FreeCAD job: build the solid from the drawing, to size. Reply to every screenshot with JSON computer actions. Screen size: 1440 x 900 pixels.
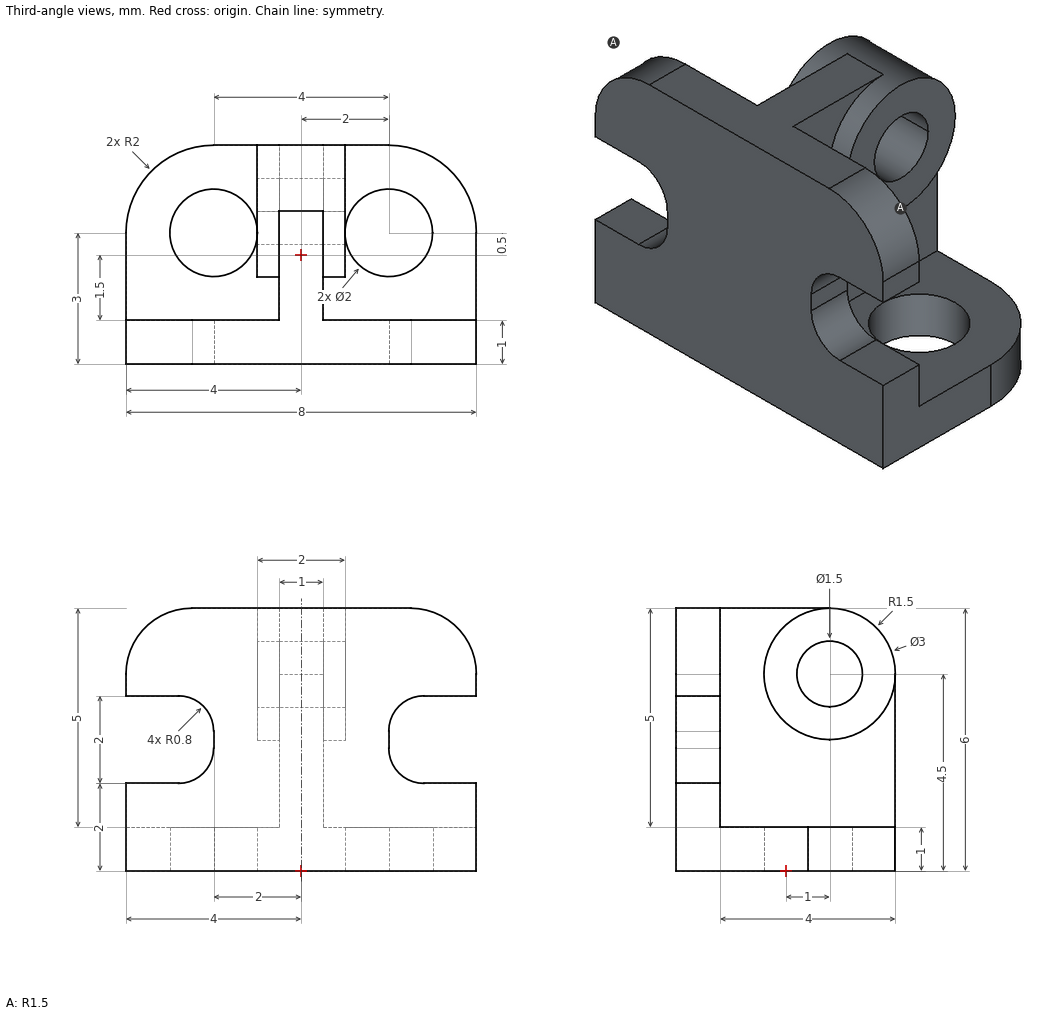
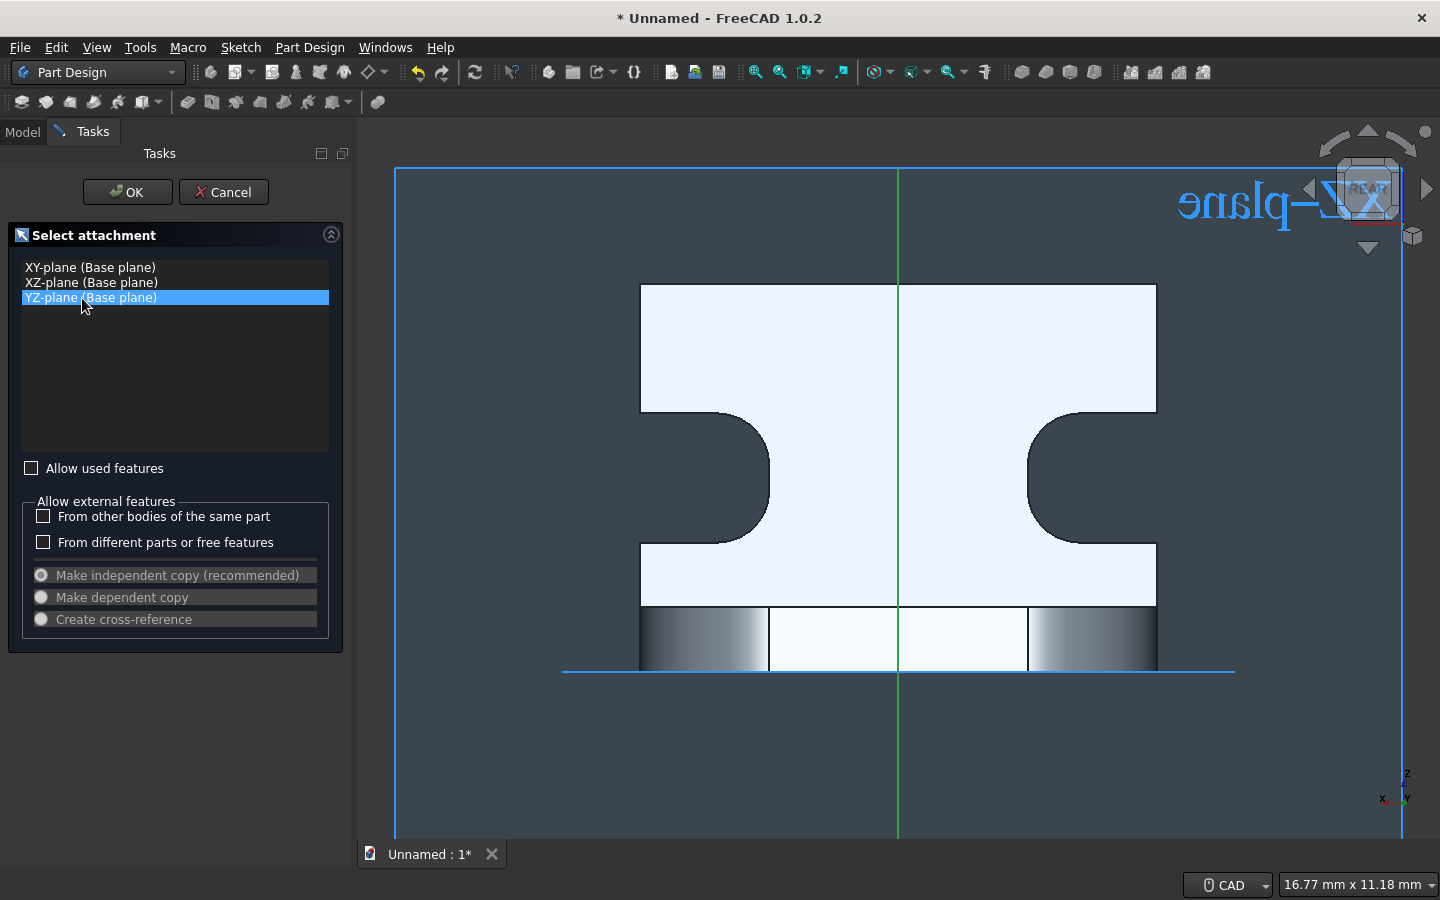
{"action": "left_click", "coordinate": [128, 192]}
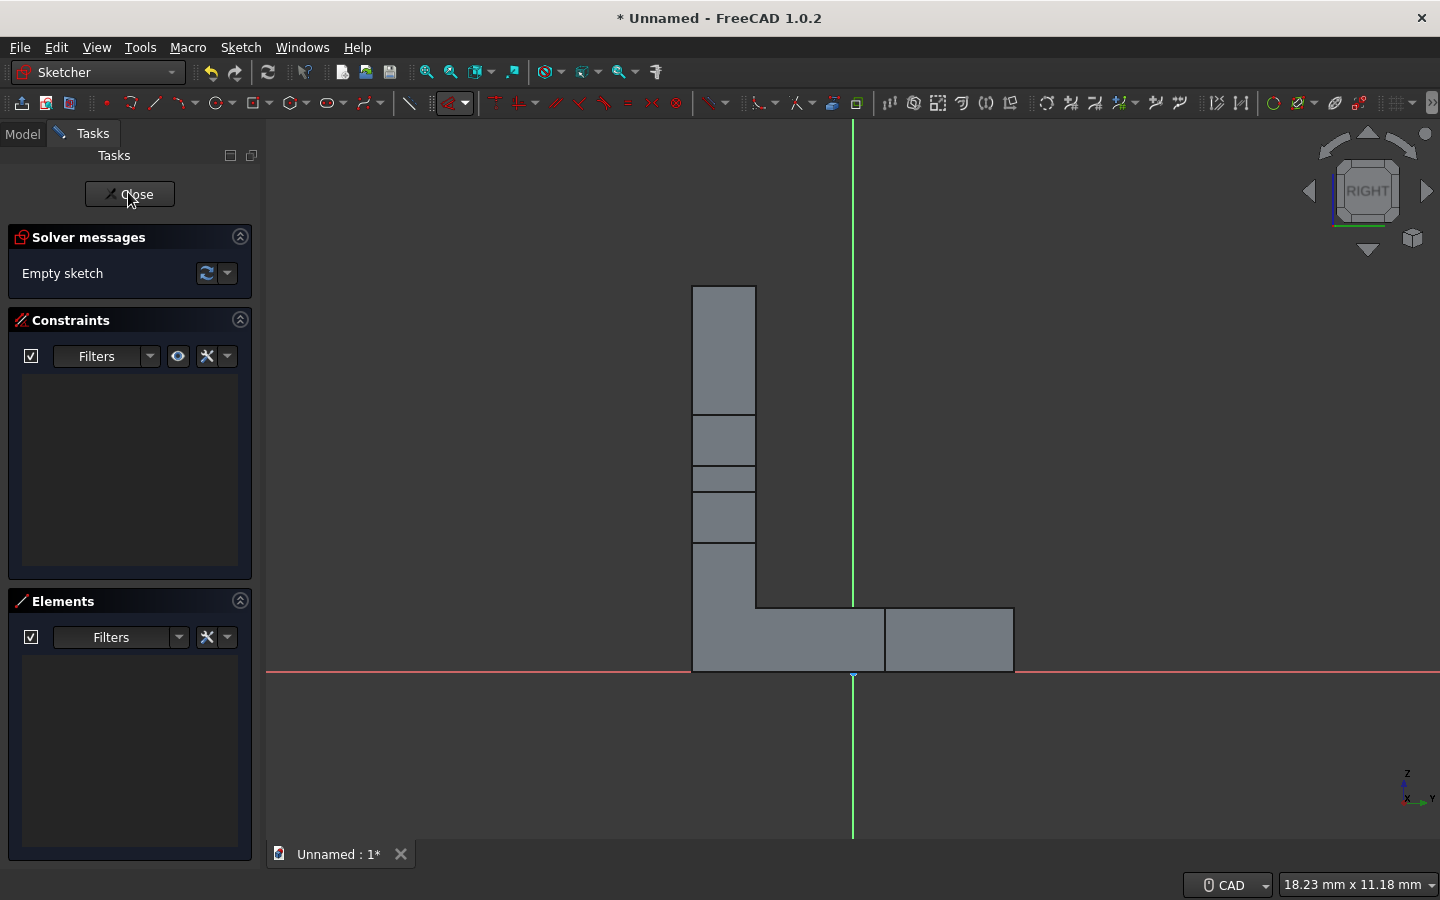
{"action": "left_click", "coordinate": [70, 104]}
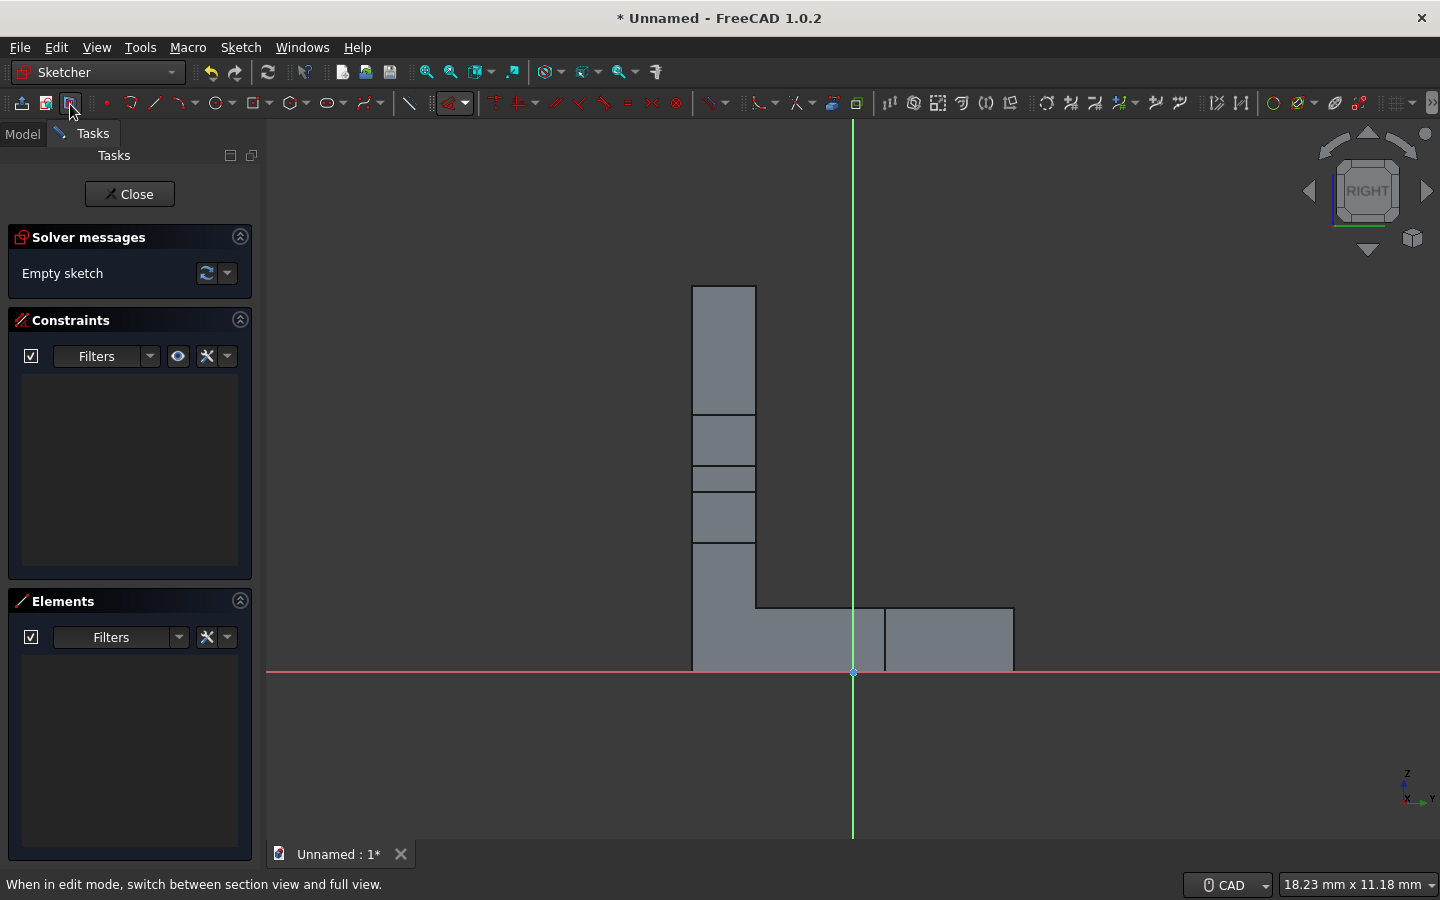
{"action": "left_click", "coordinate": [132, 104]}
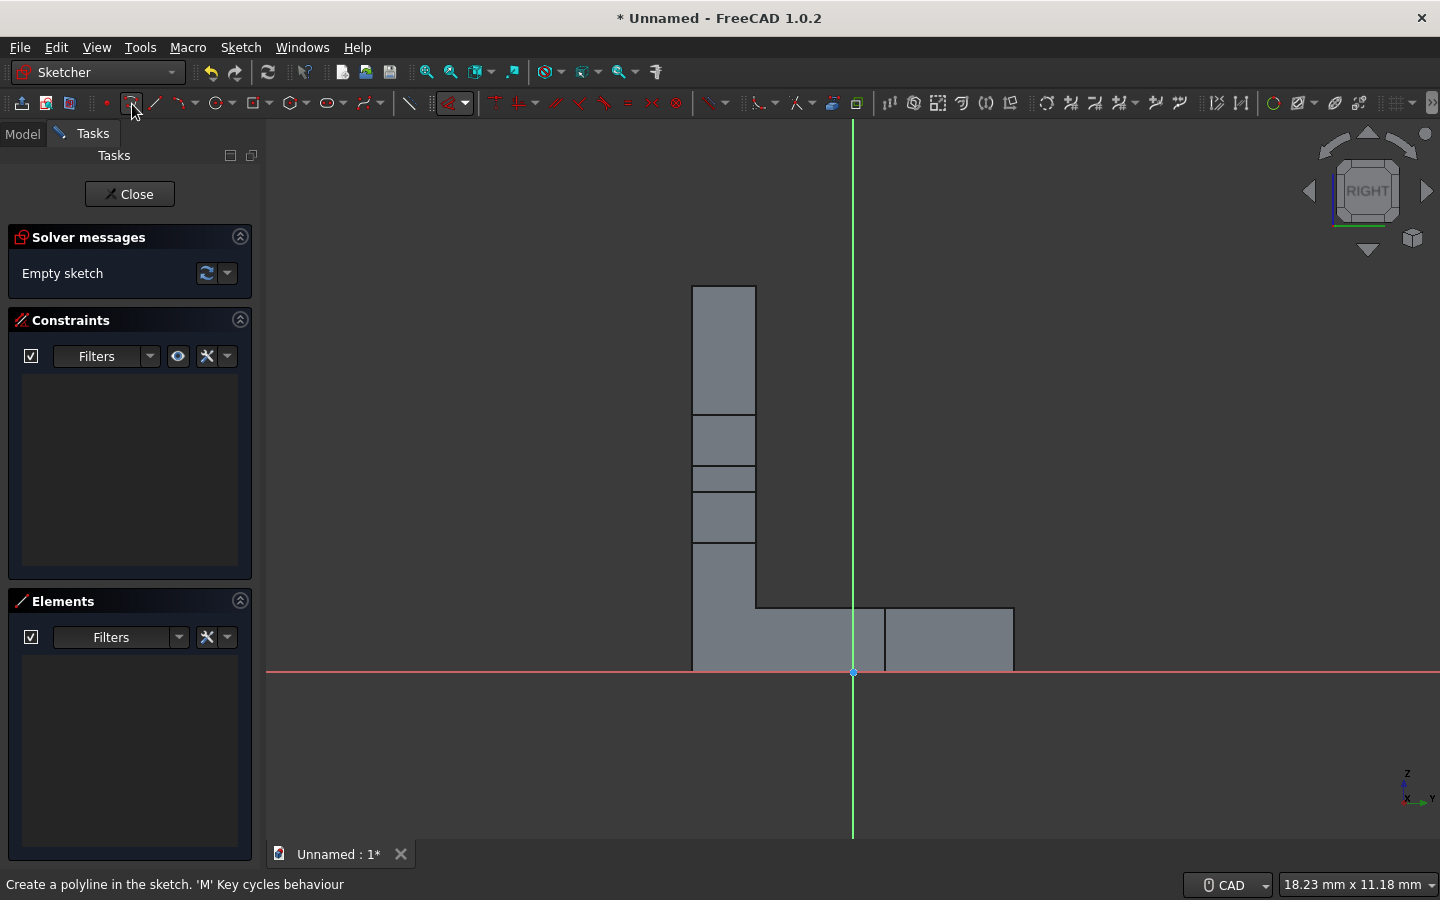
{"action": "left_click", "coordinate": [917, 286]}
{"action": "left_click", "coordinate": [756, 286]}
{"action": "left_click", "coordinate": [756, 608]}
{"action": "left_click", "coordinate": [1014, 608]}
{"action": "left_click", "coordinate": [1014, 382]}
{"action": "right_click", "coordinate": [1014, 382]}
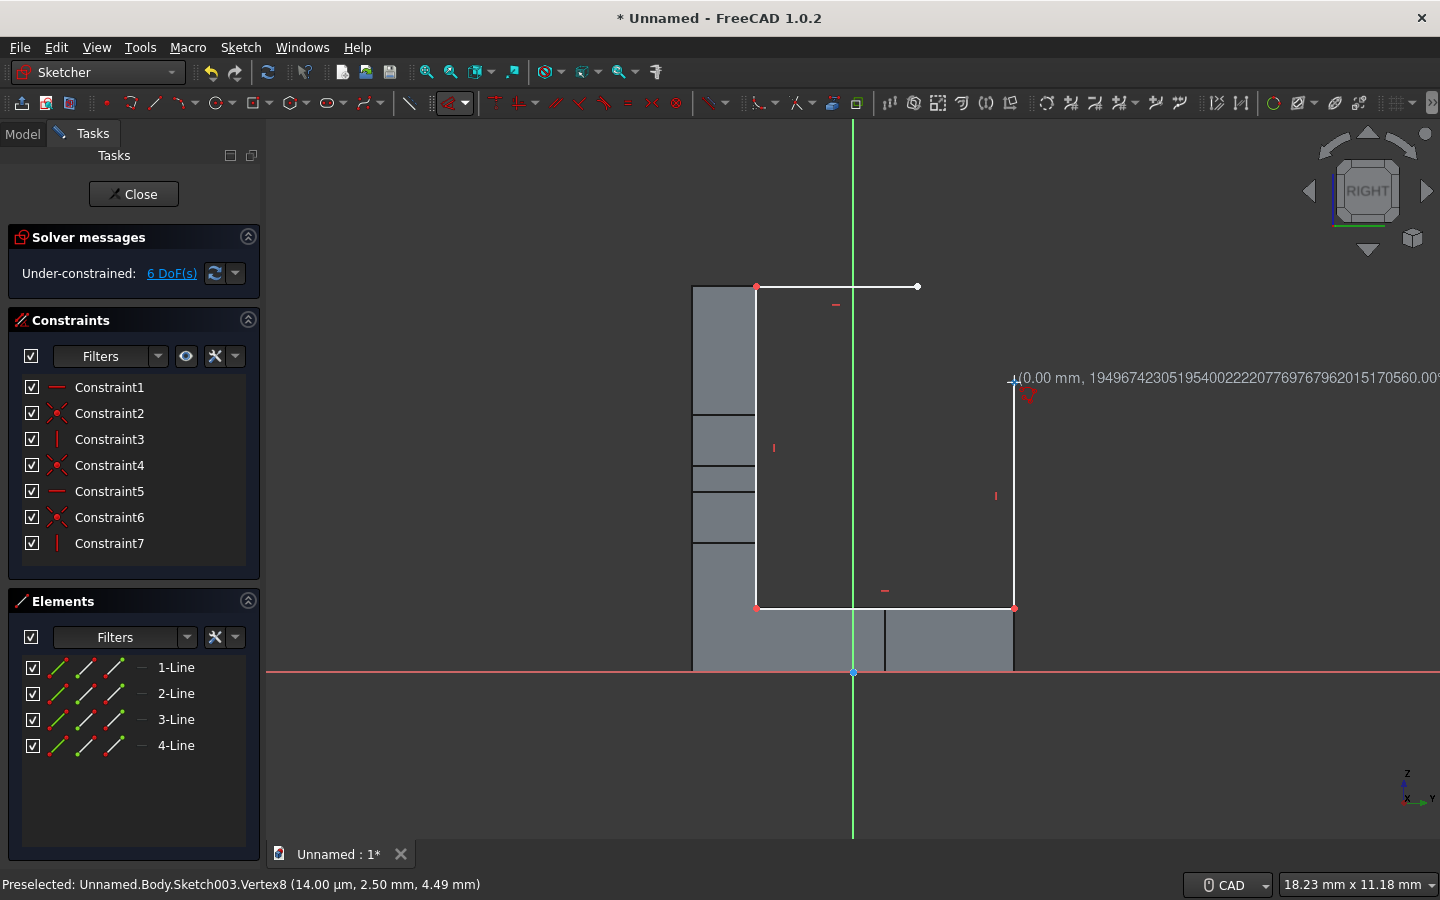
{"action": "left_click", "coordinate": [180, 104]}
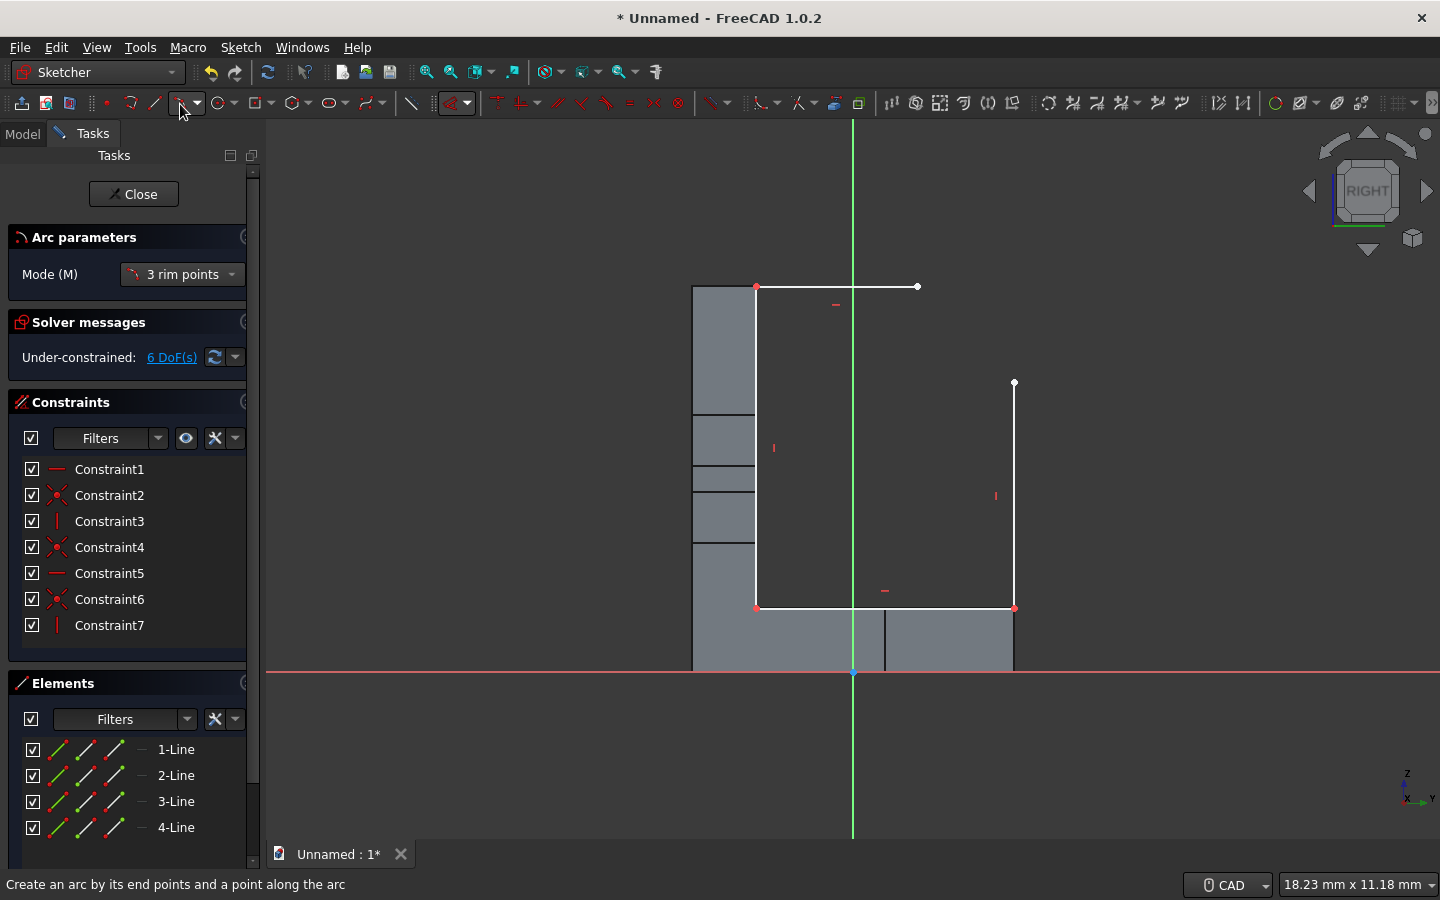
{"action": "left_click", "coordinate": [1014, 383]}
{"action": "left_click", "coordinate": [917, 287]}
{"action": "left_click", "coordinate": [986, 314]}
{"action": "key", "text": "Escape"}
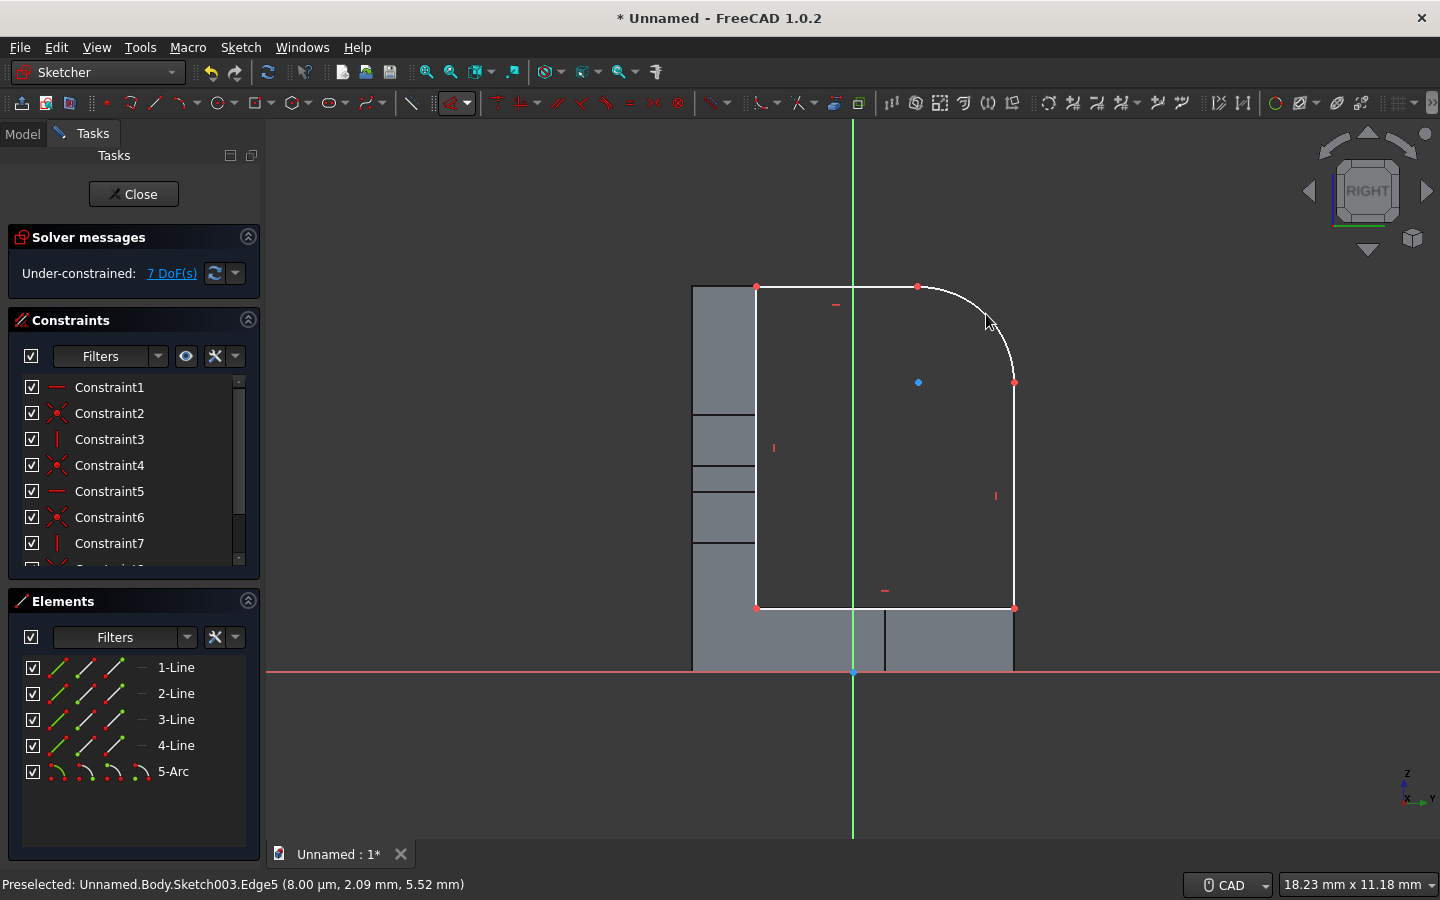
{"action": "left_click", "coordinate": [869, 287]}